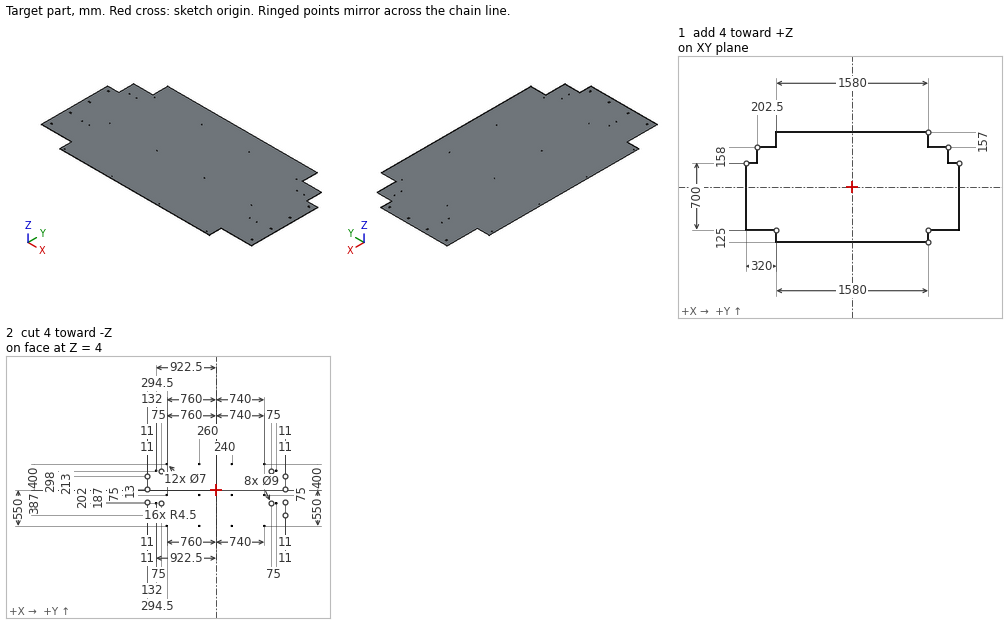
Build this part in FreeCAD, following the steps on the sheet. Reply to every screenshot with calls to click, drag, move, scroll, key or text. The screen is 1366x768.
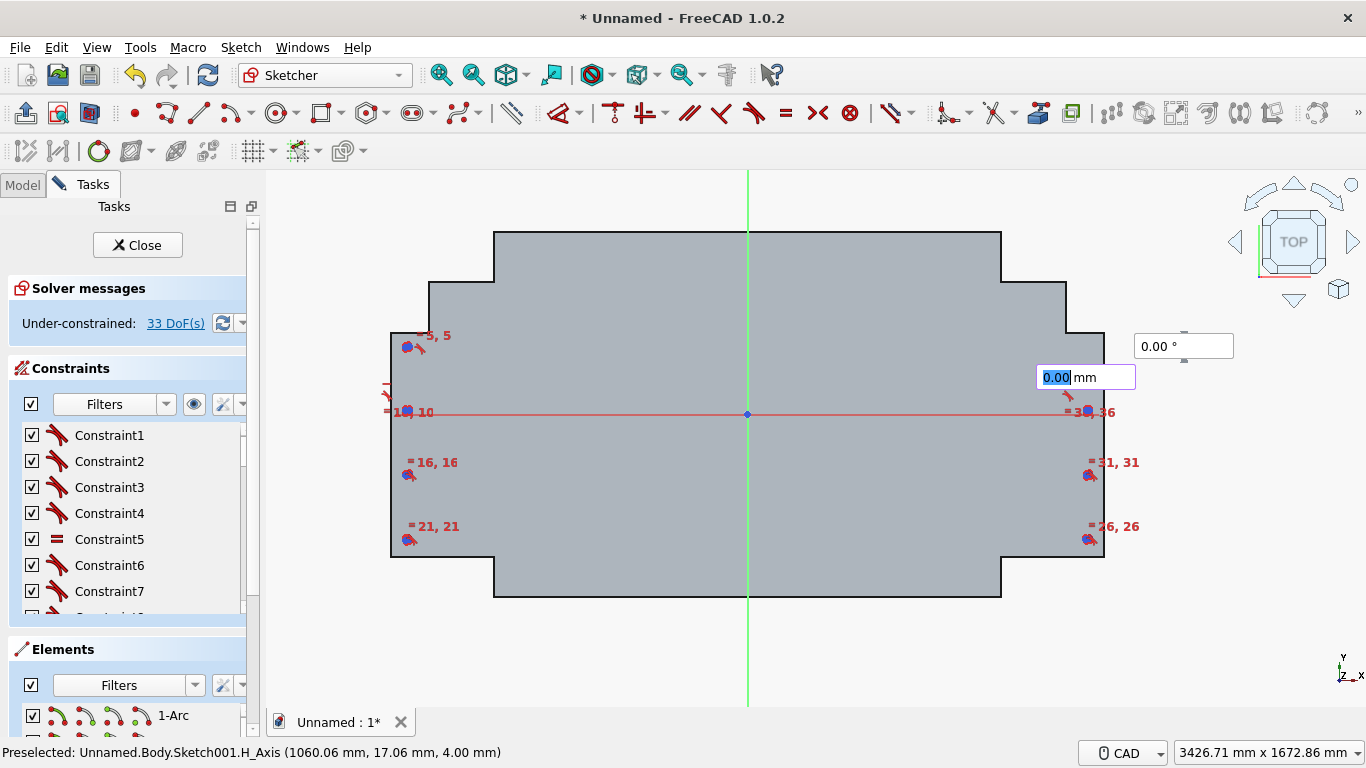
scroll(1090, 346, up, 8)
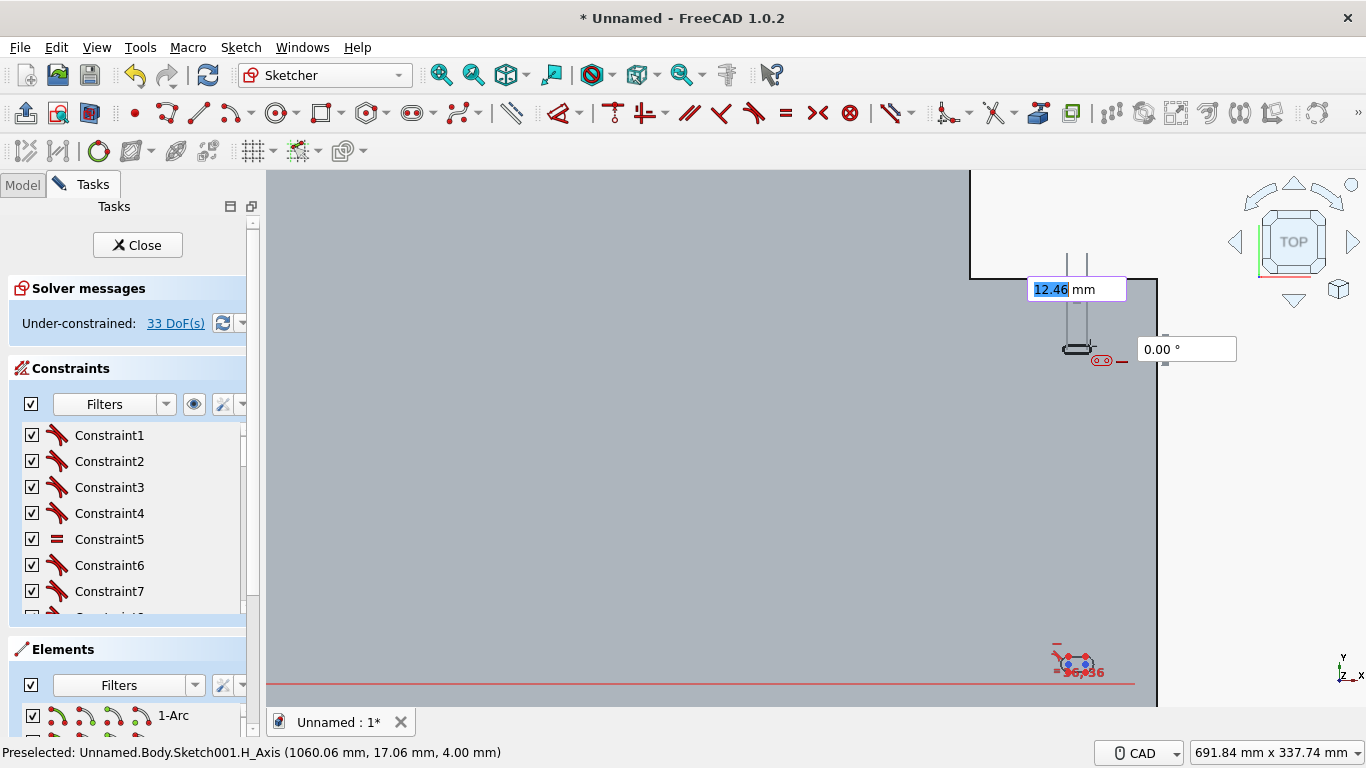
click(1086, 345)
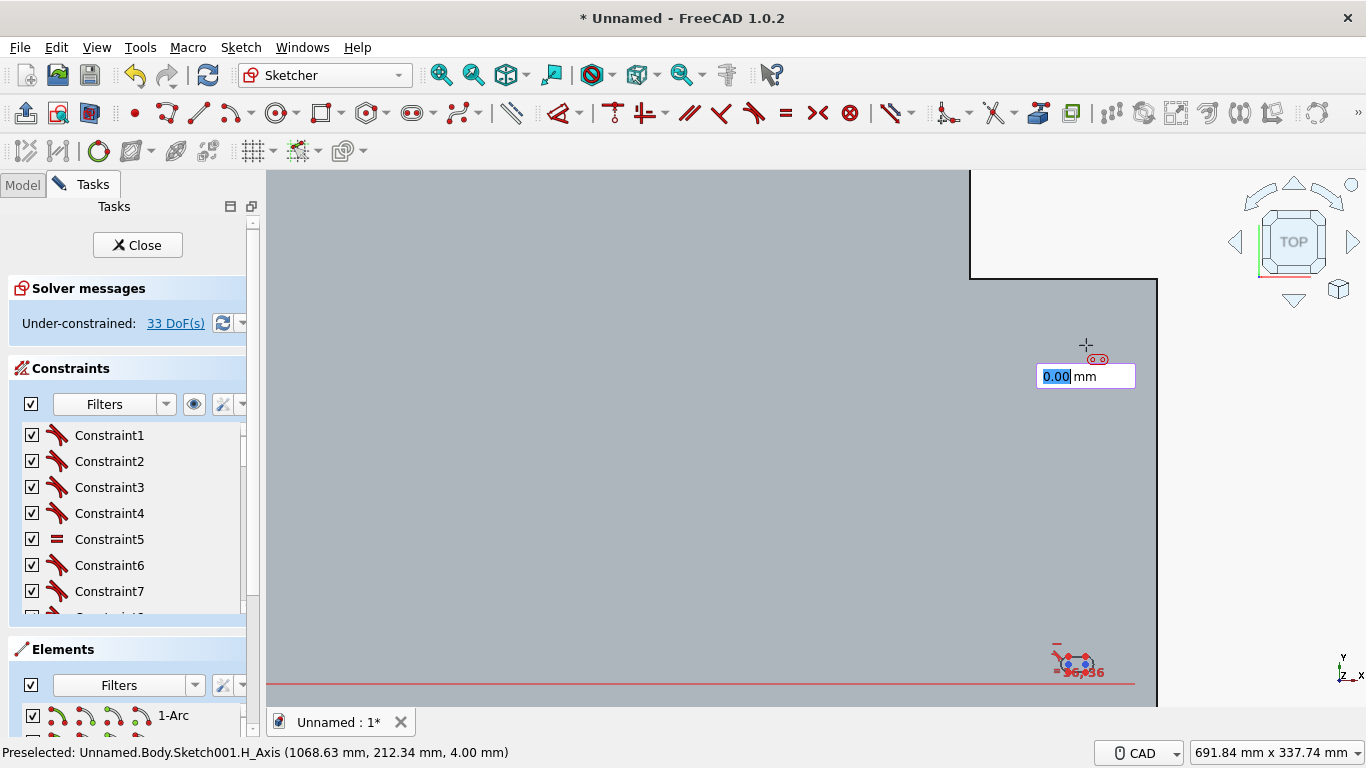
scroll(1077, 338, up, 4)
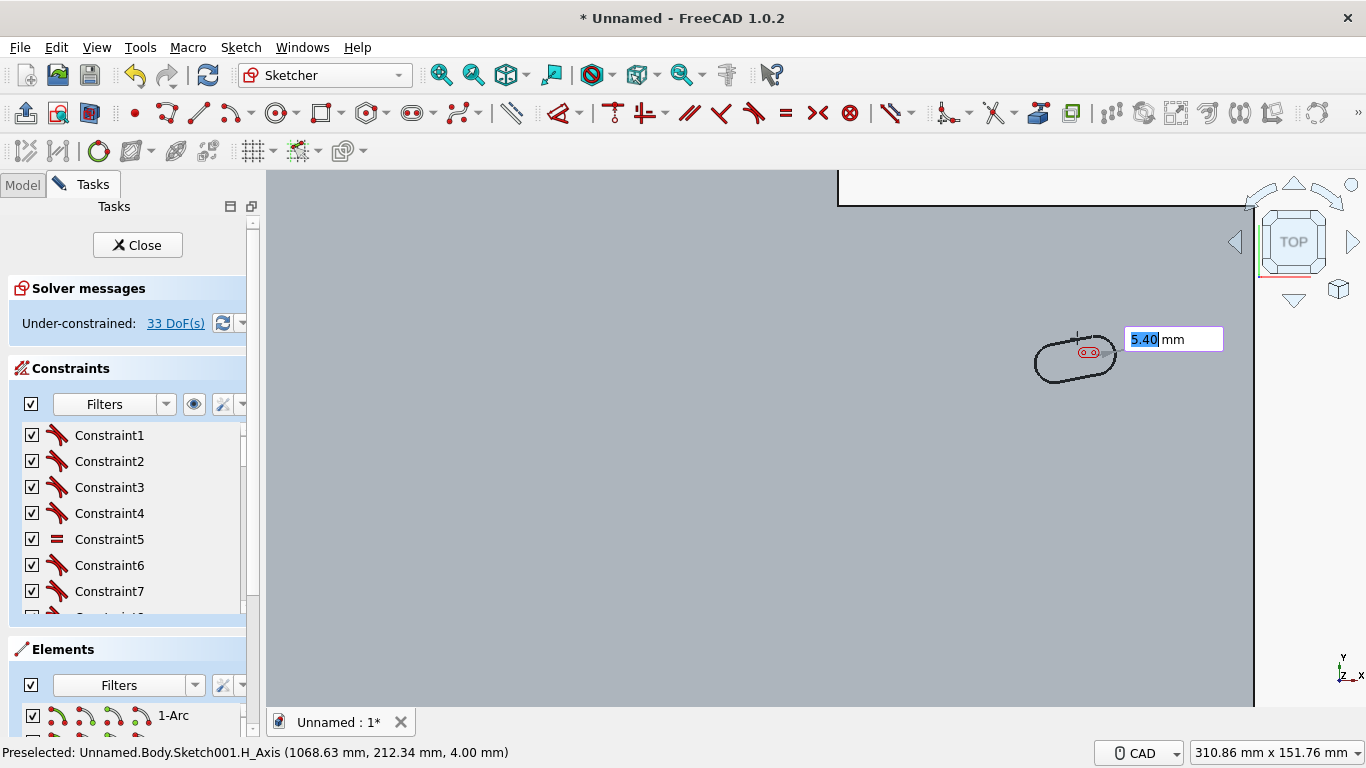
click(1077, 338)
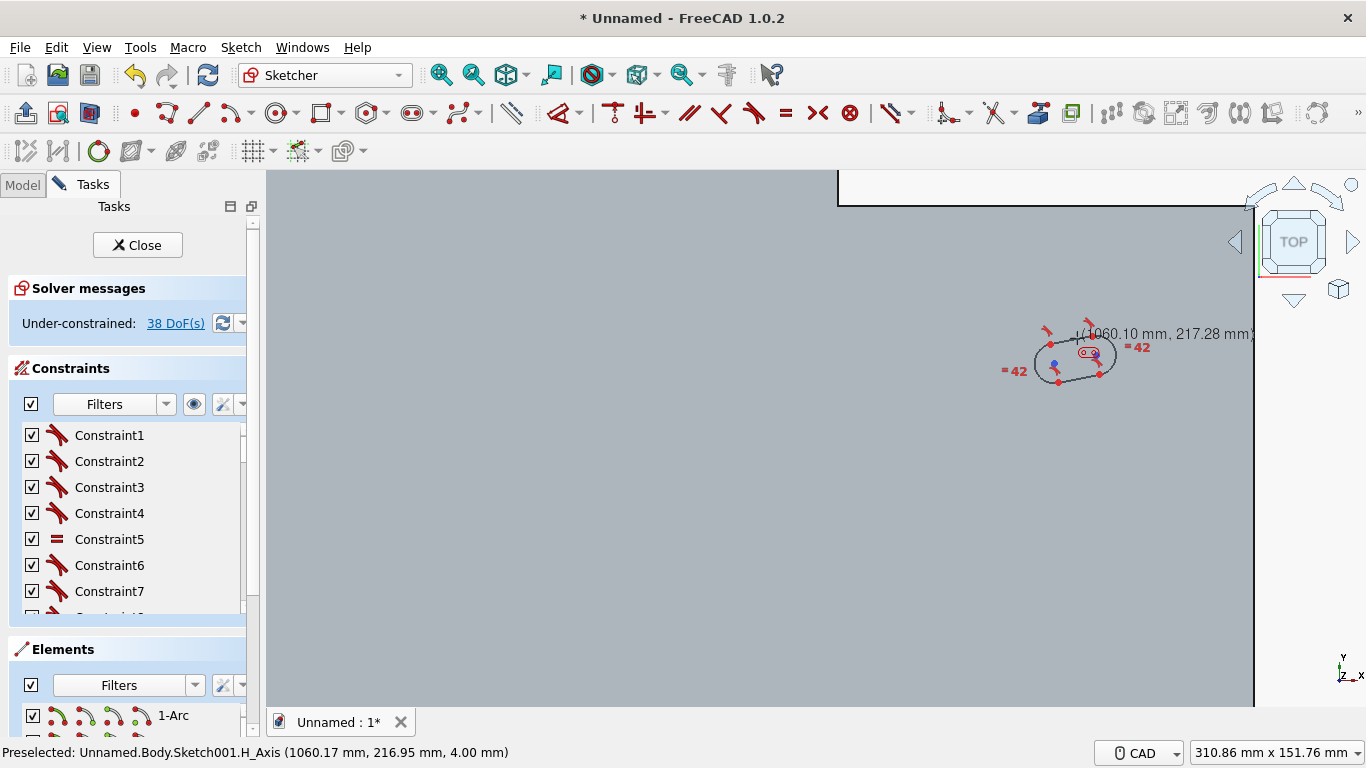
click(276, 114)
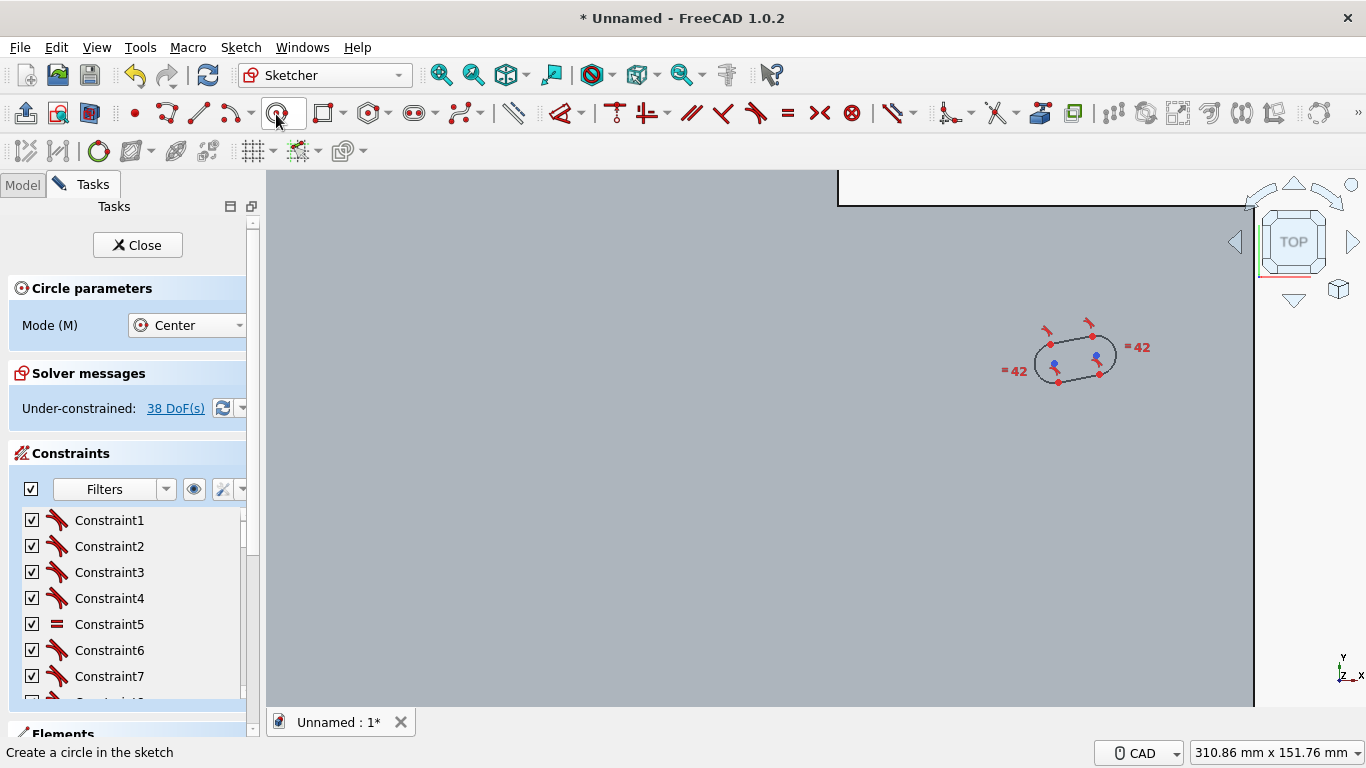
scroll(1089, 345, down, 12)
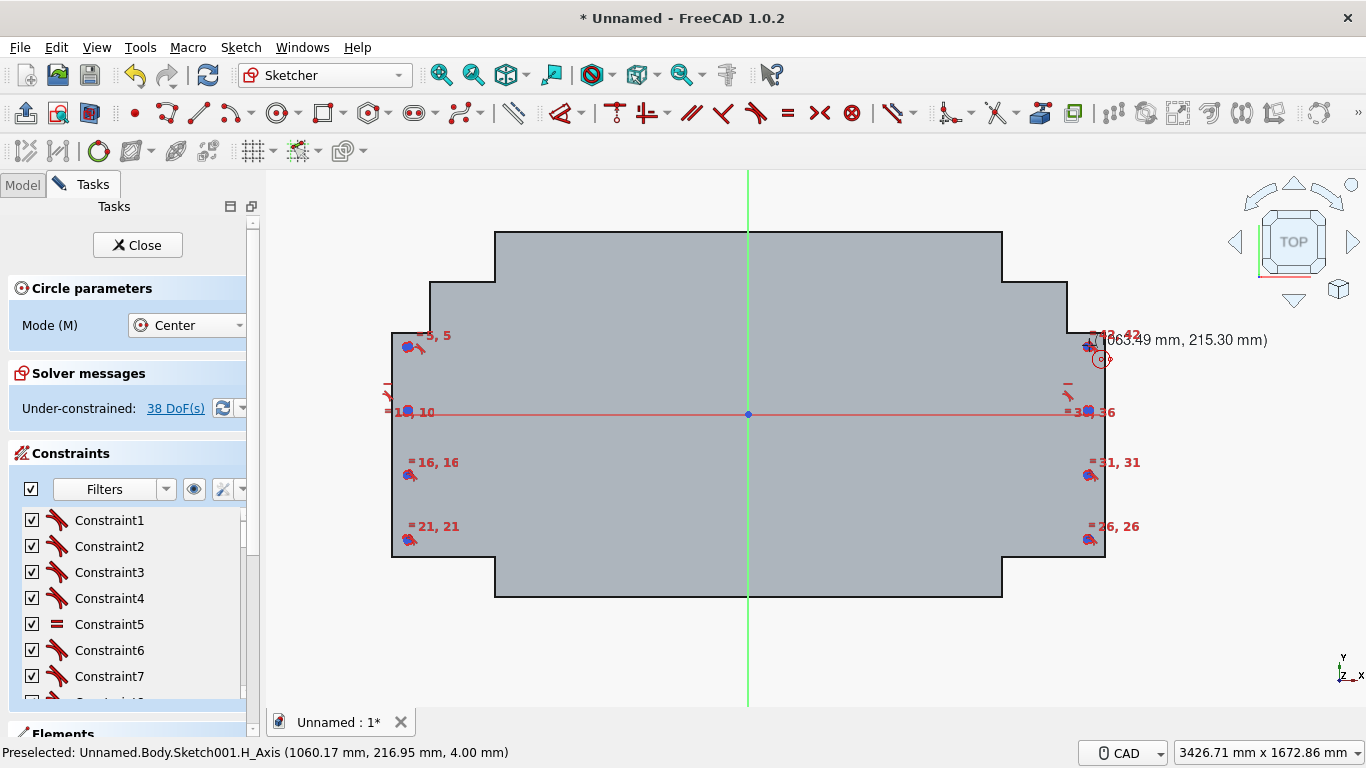
scroll(504, 286, up, 16)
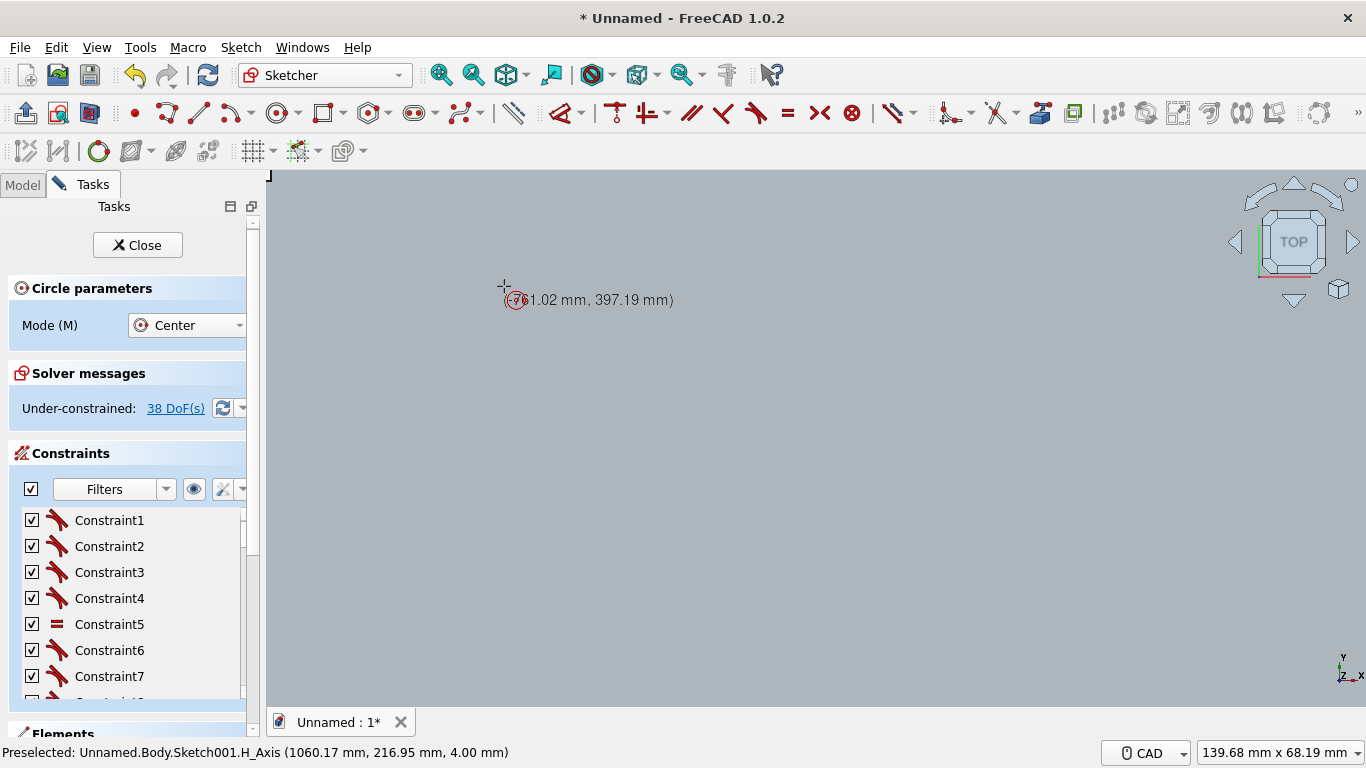
scroll(447, 251, down, 15)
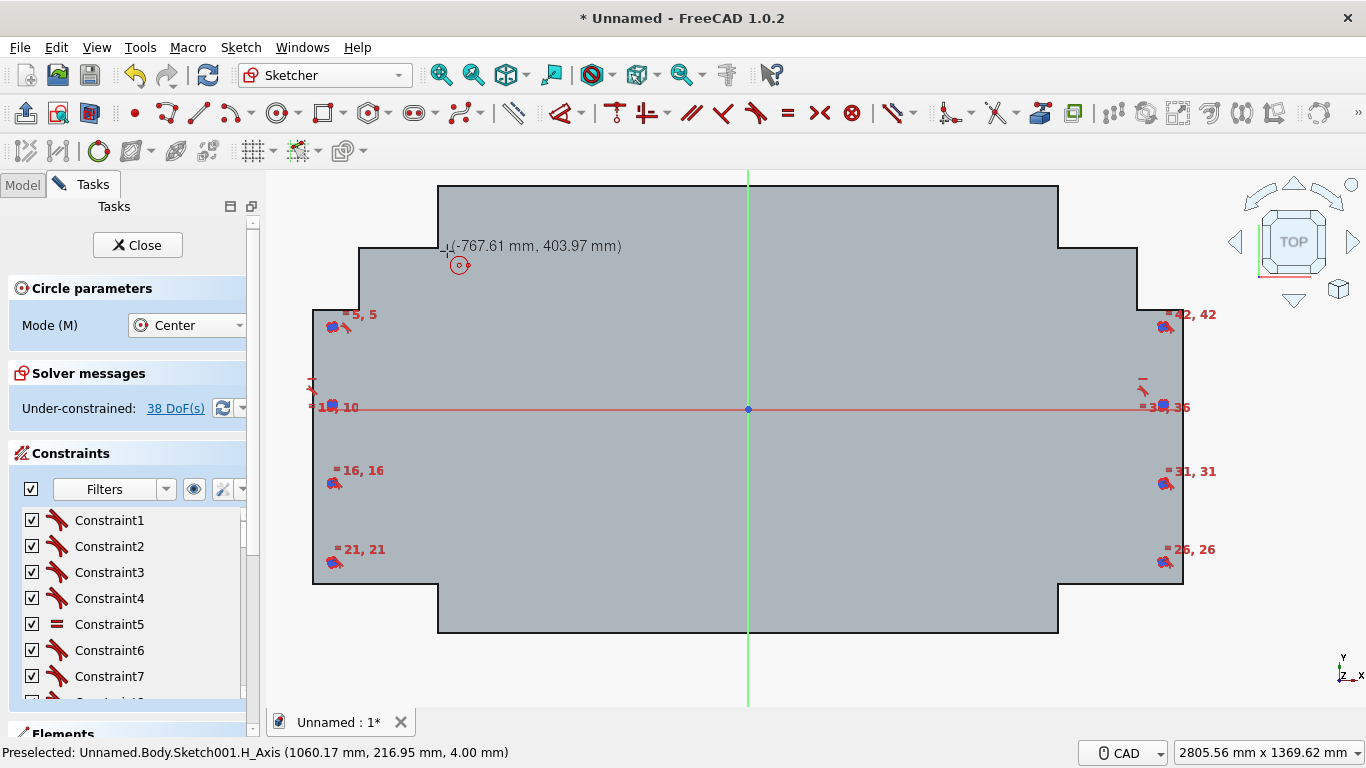
click(450, 253)
move(451, 252)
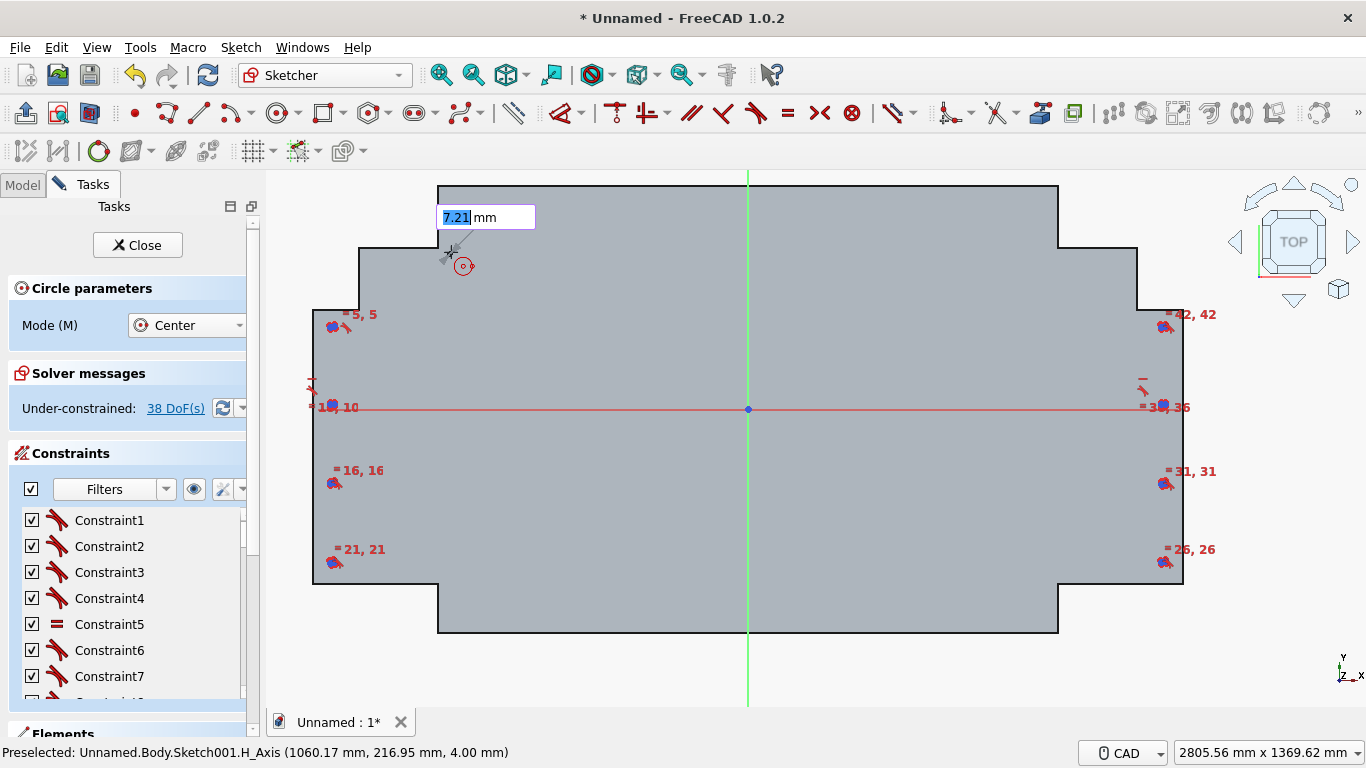
text(7)
key(Return)